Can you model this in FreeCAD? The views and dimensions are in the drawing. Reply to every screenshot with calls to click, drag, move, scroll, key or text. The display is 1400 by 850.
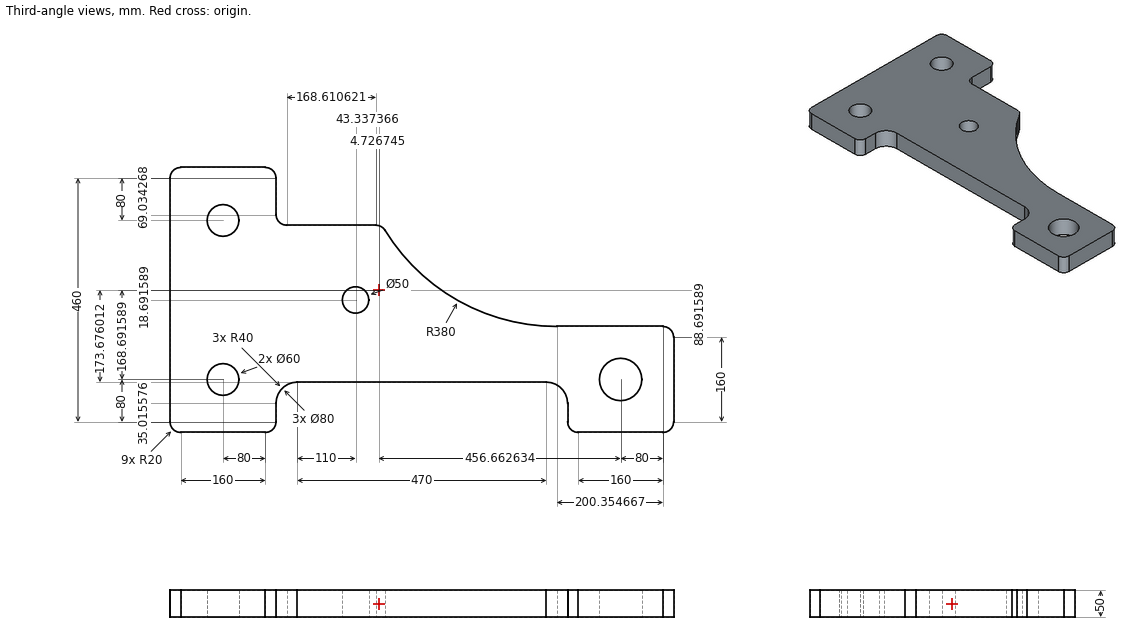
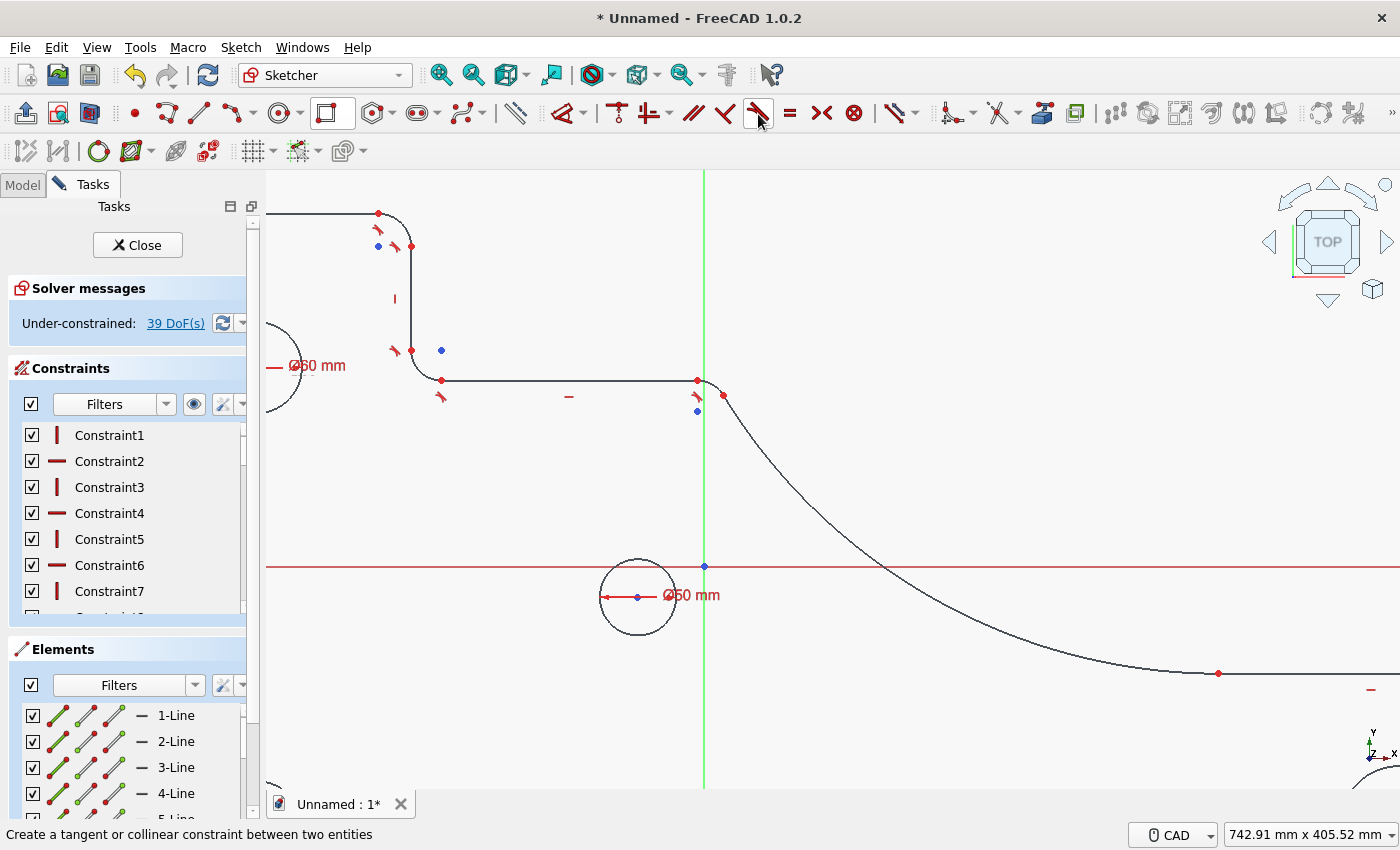
click(305, 214)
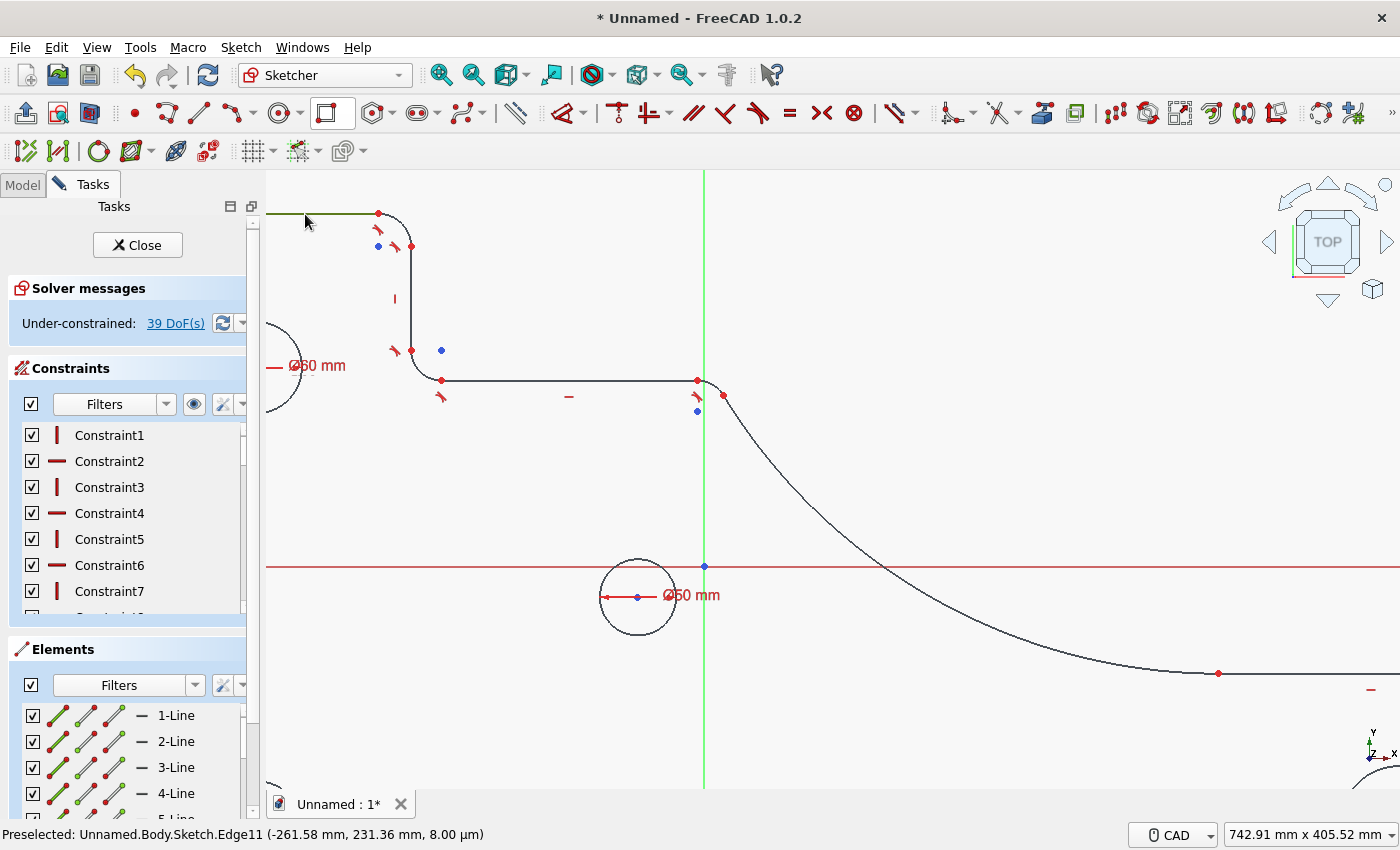
scroll(712, 385, down, 4)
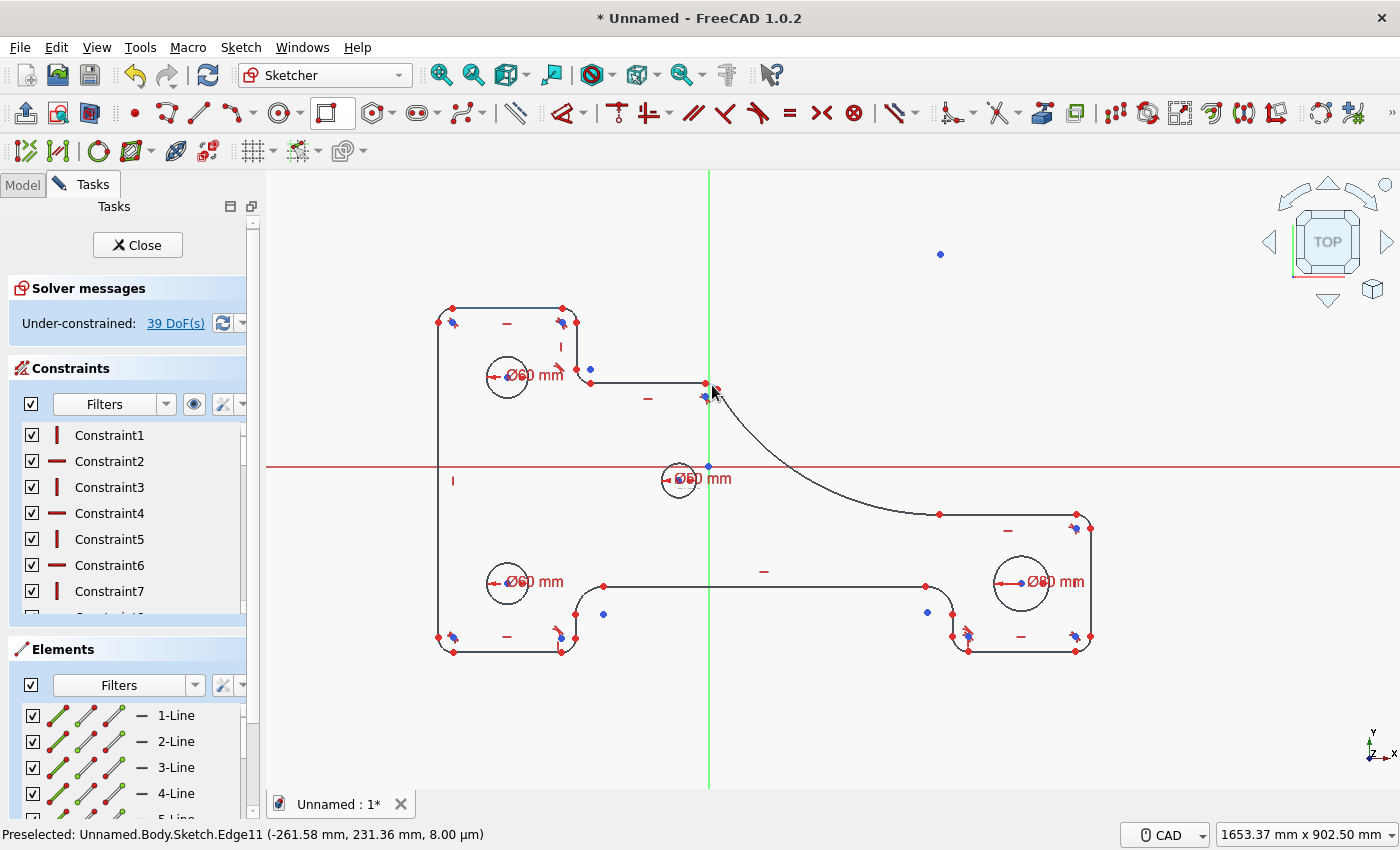
scroll(446, 310, up, 4)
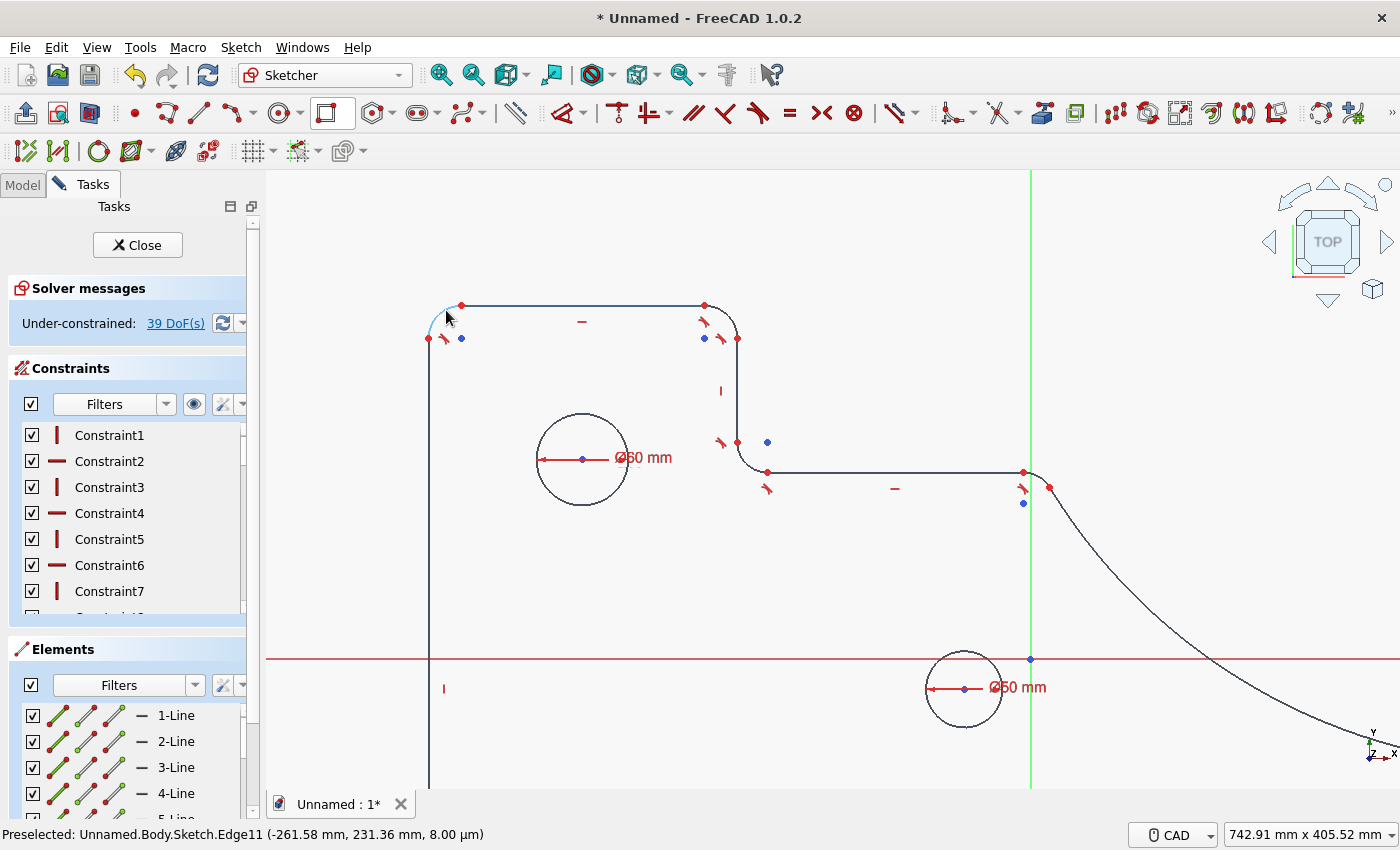
click(446, 309)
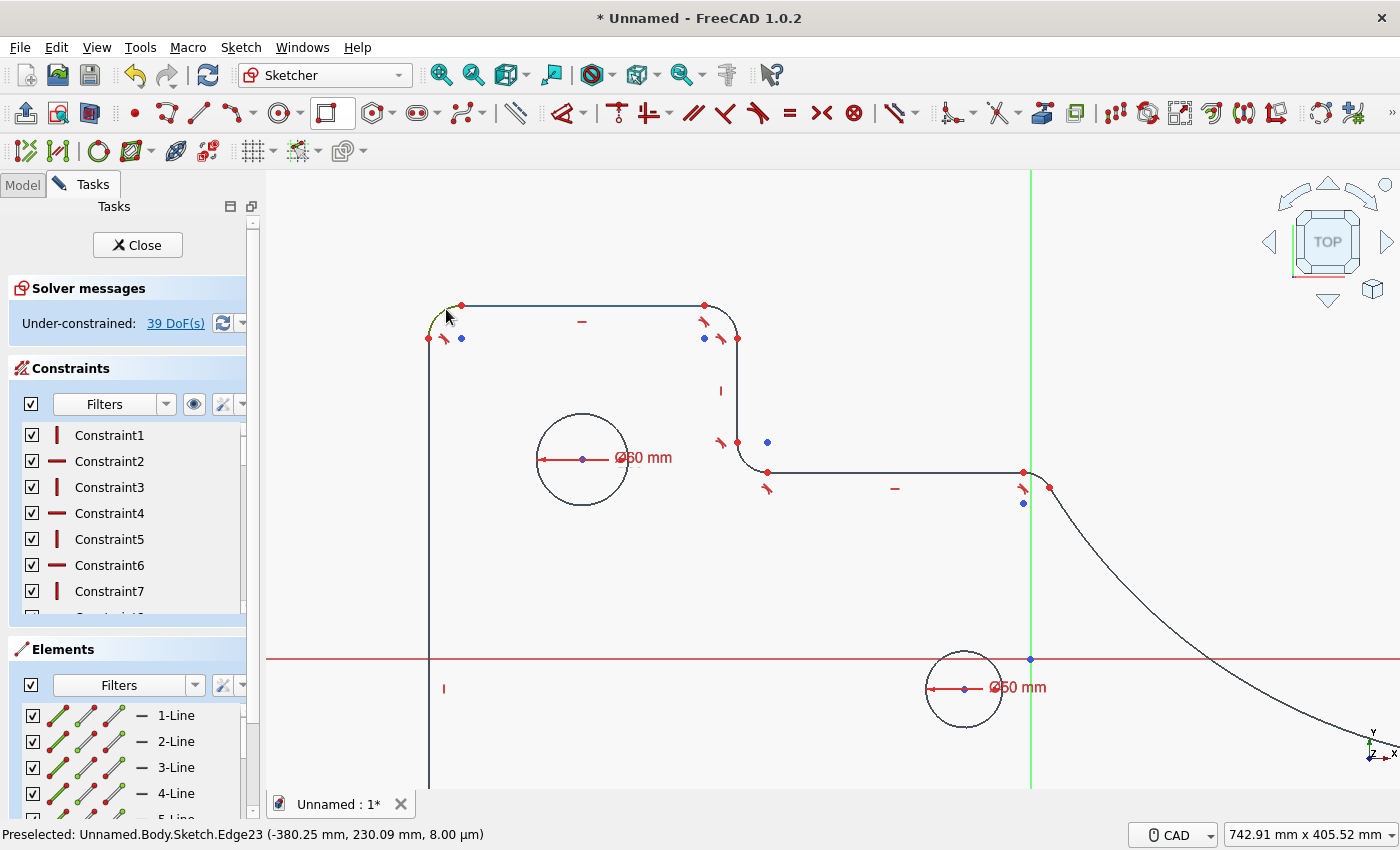
click(758, 114)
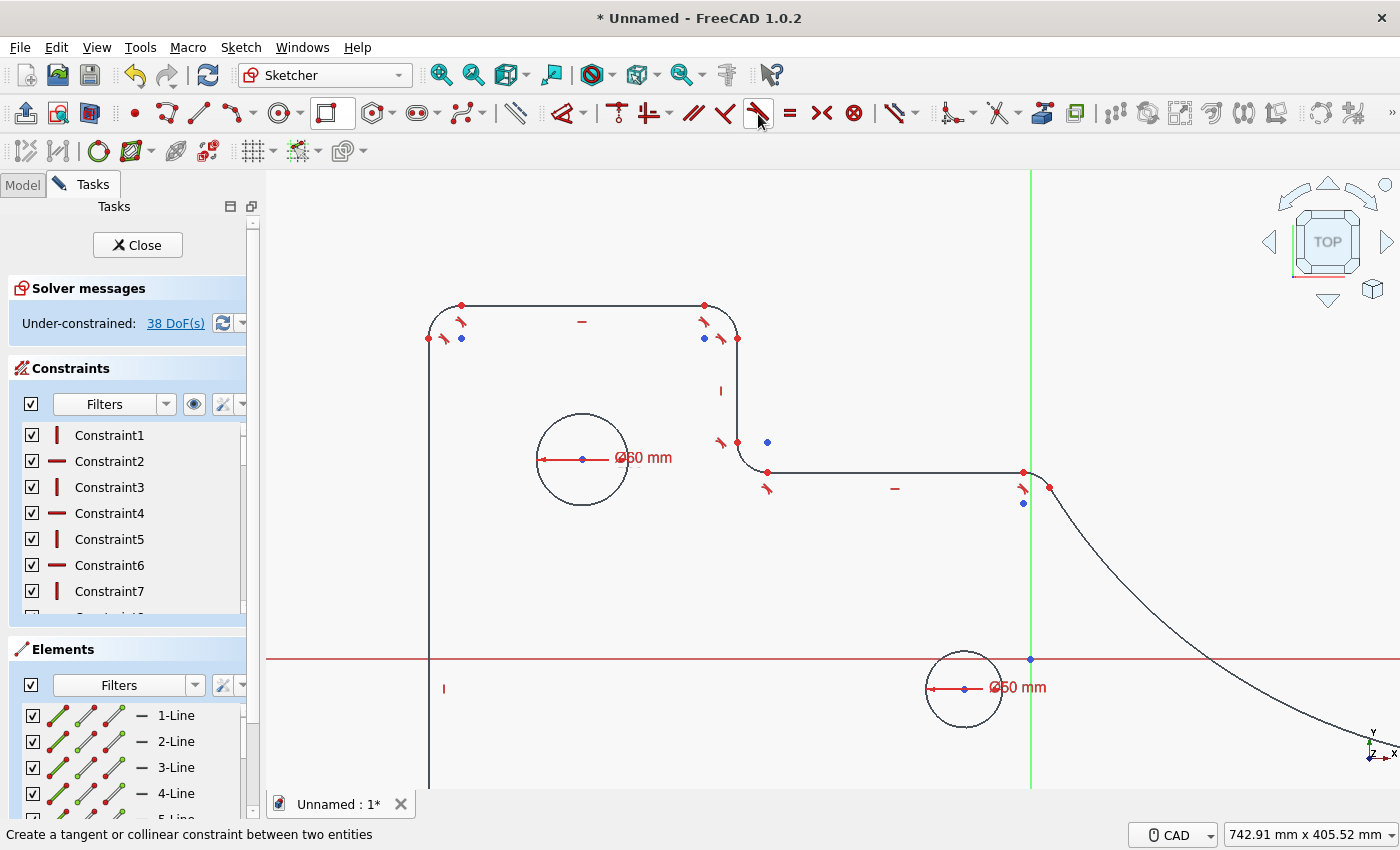
click(1164, 623)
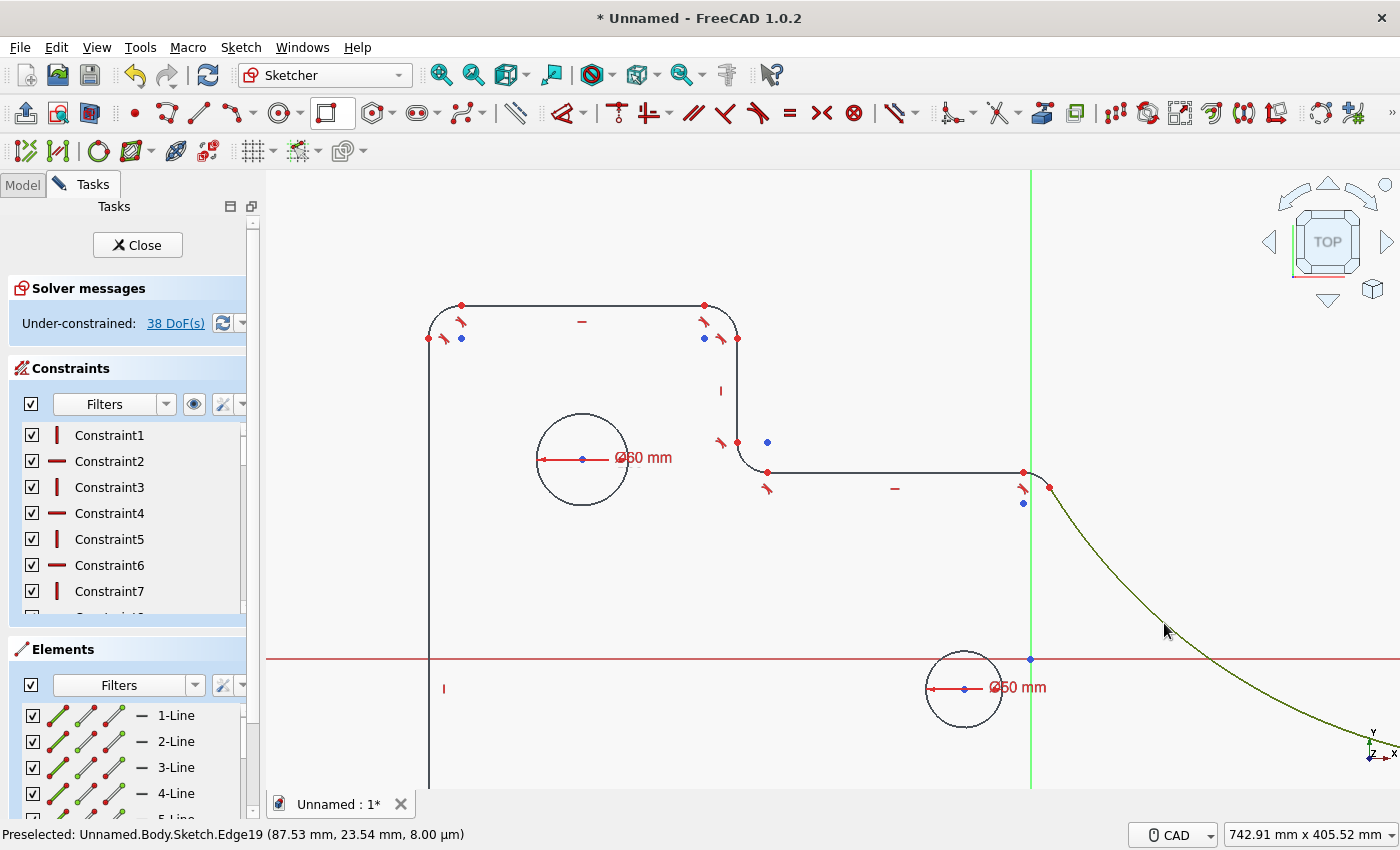
scroll(1044, 480, up, 2)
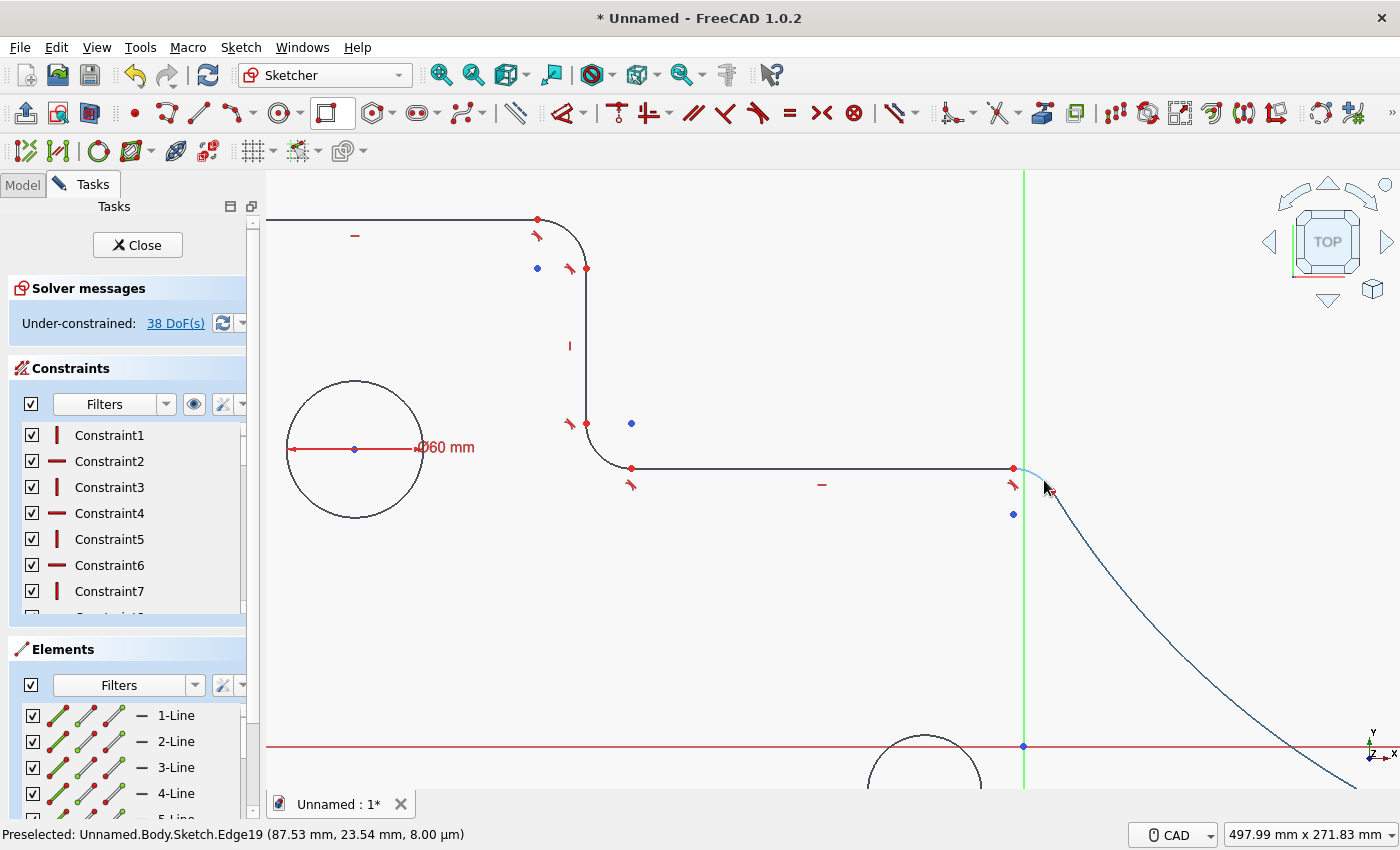
click(1043, 480)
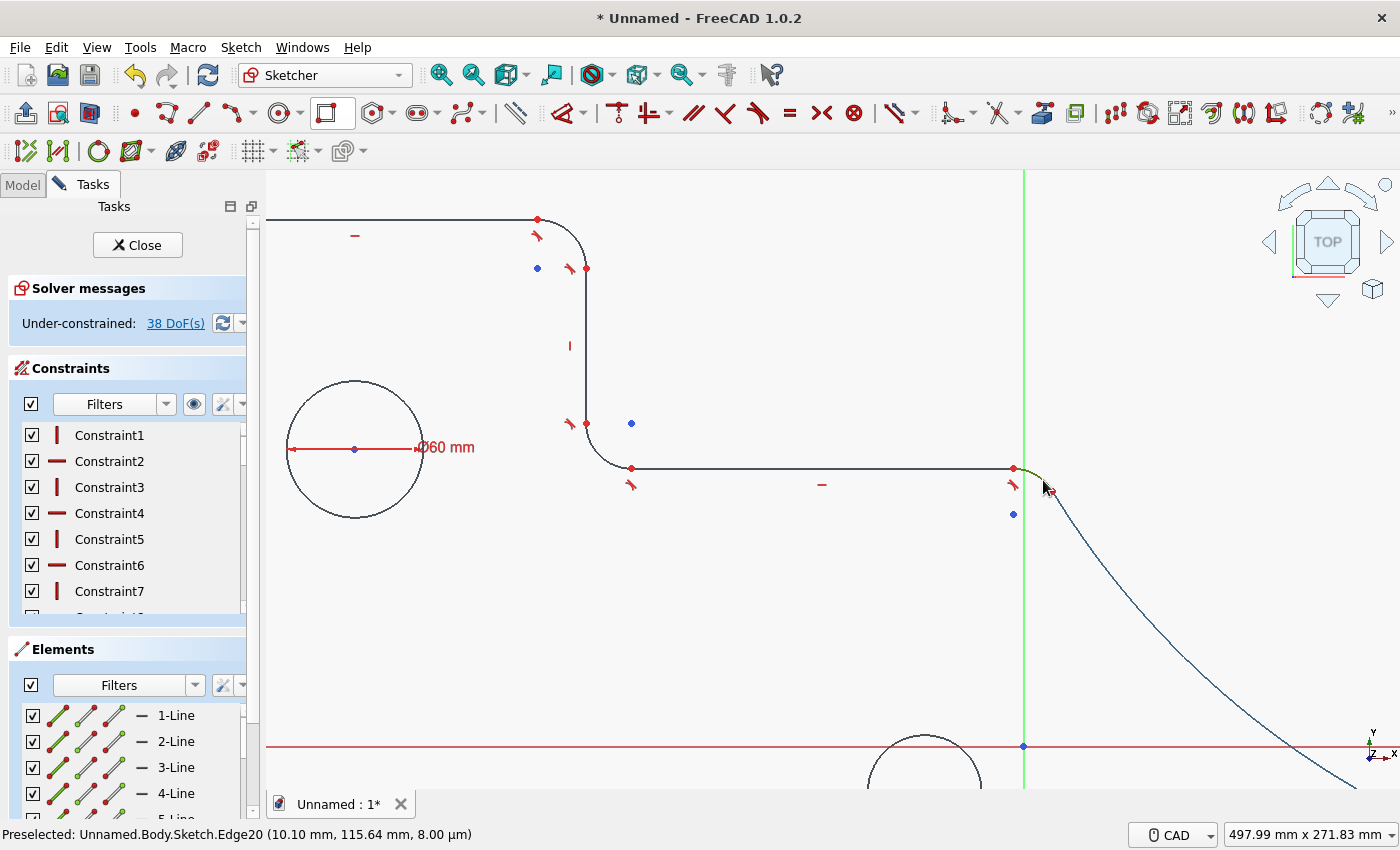
click(758, 114)